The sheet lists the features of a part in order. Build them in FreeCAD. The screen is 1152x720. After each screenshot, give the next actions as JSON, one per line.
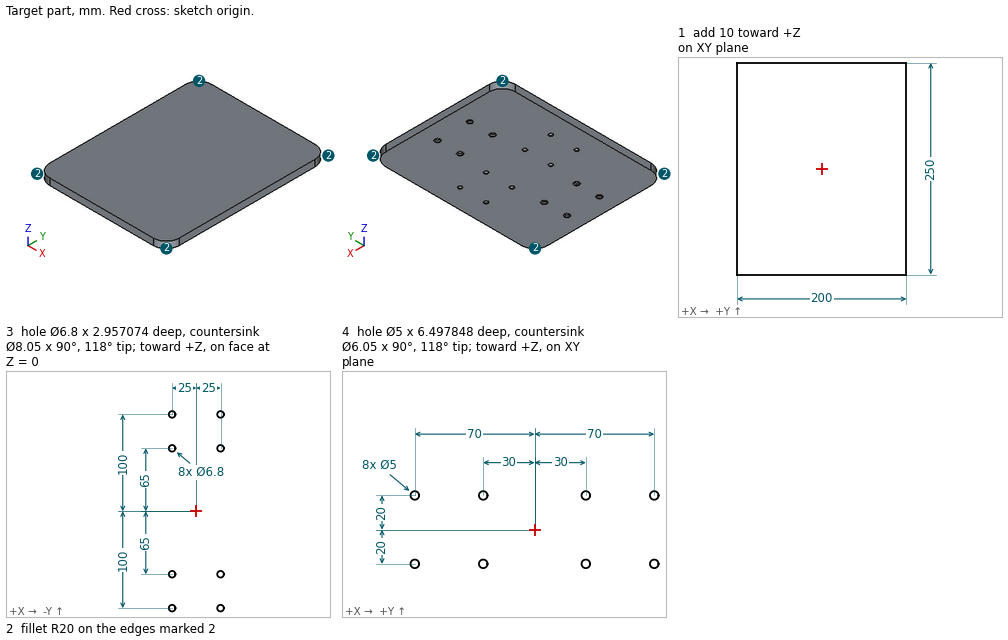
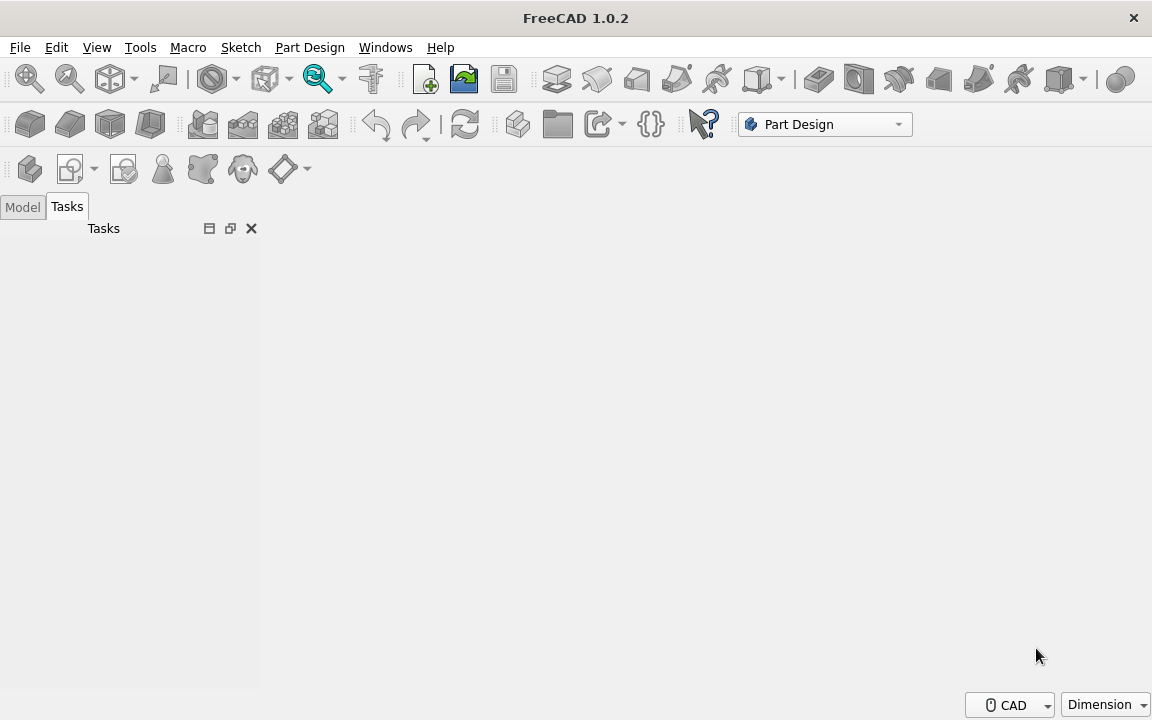
{"action": "left_click", "coordinate": [424, 80]}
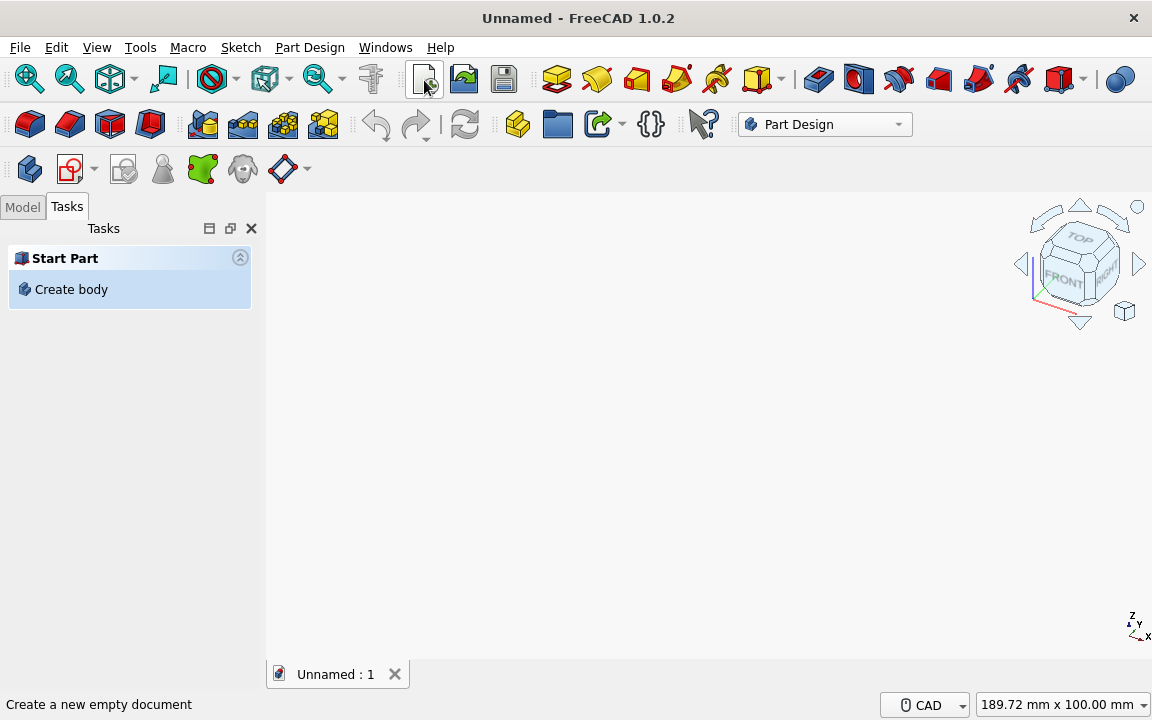
{"action": "left_click", "coordinate": [70, 170]}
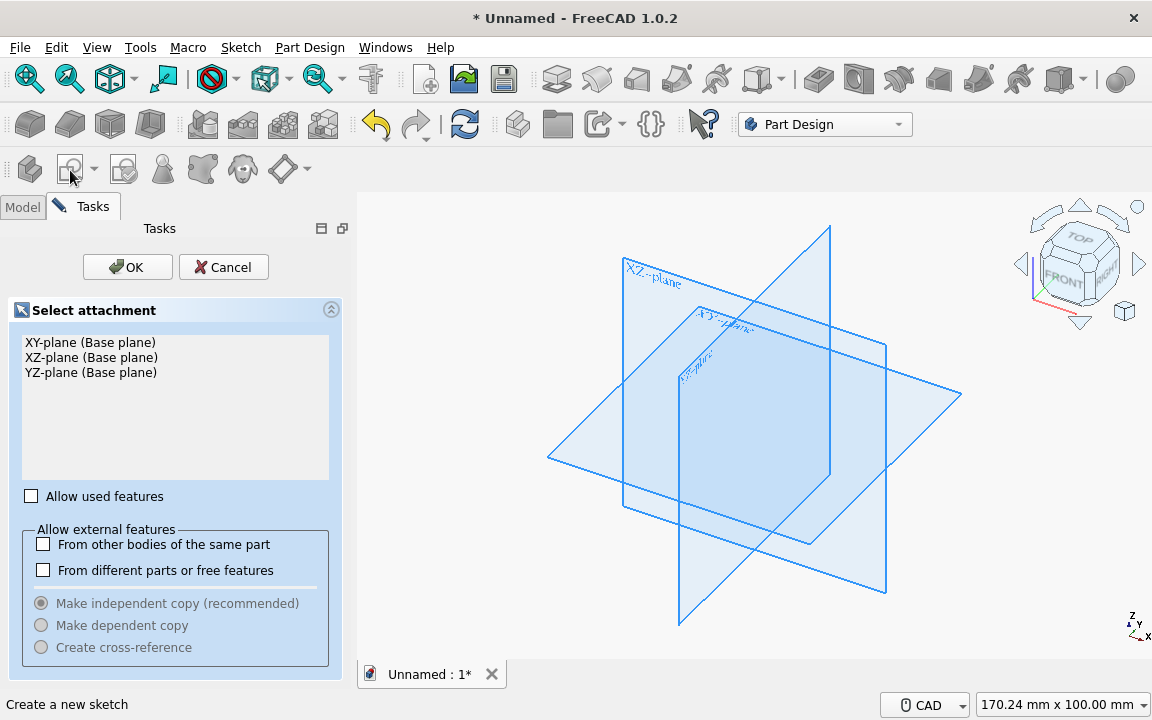
{"action": "left_click", "coordinate": [82, 342]}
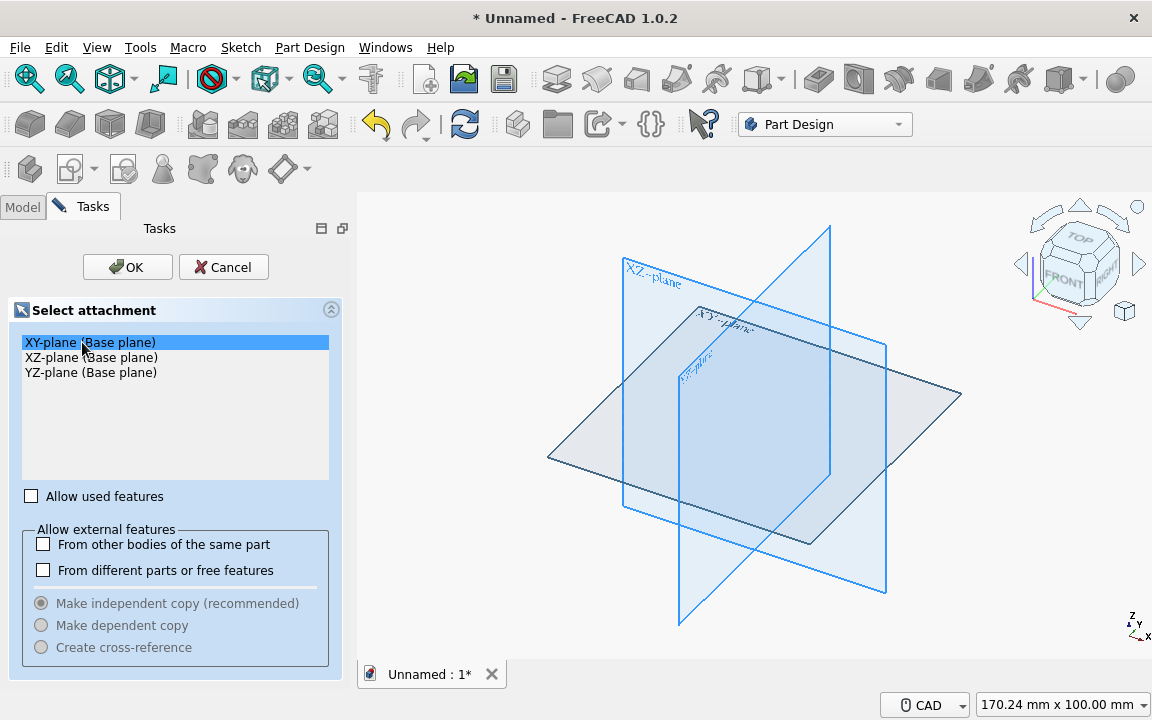
{"action": "left_click", "coordinate": [128, 267]}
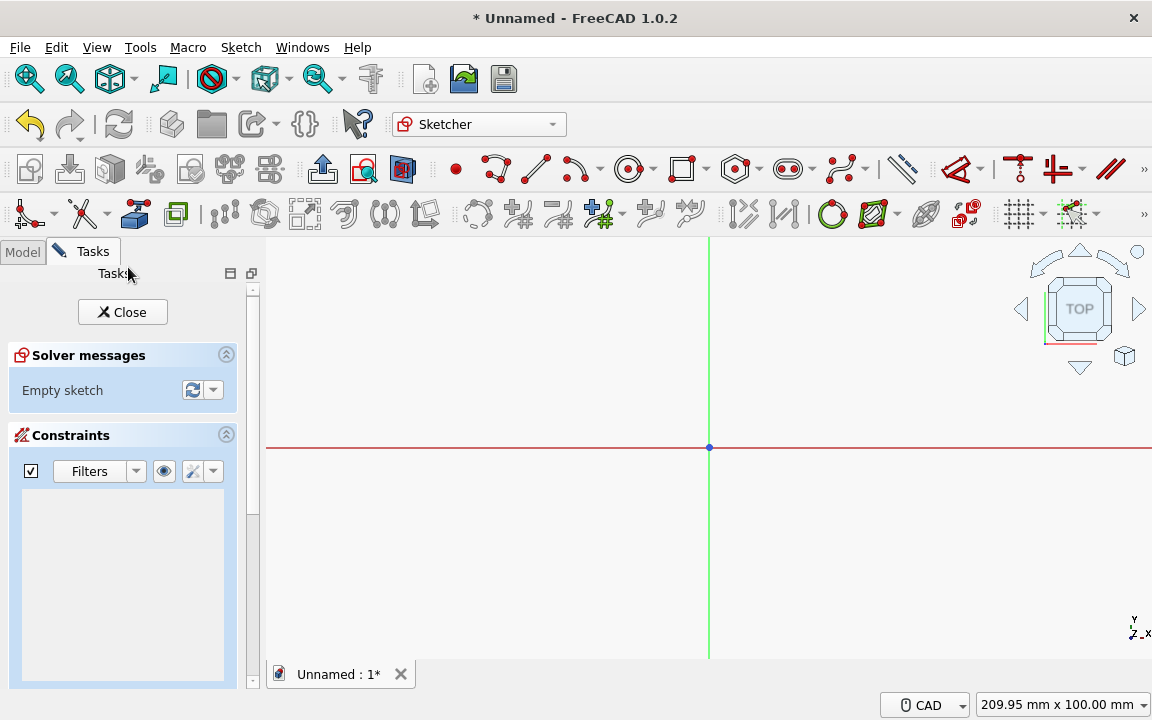
{"action": "scroll", "coordinate": [618, 448], "scroll_direction": "down", "scroll_amount": 7}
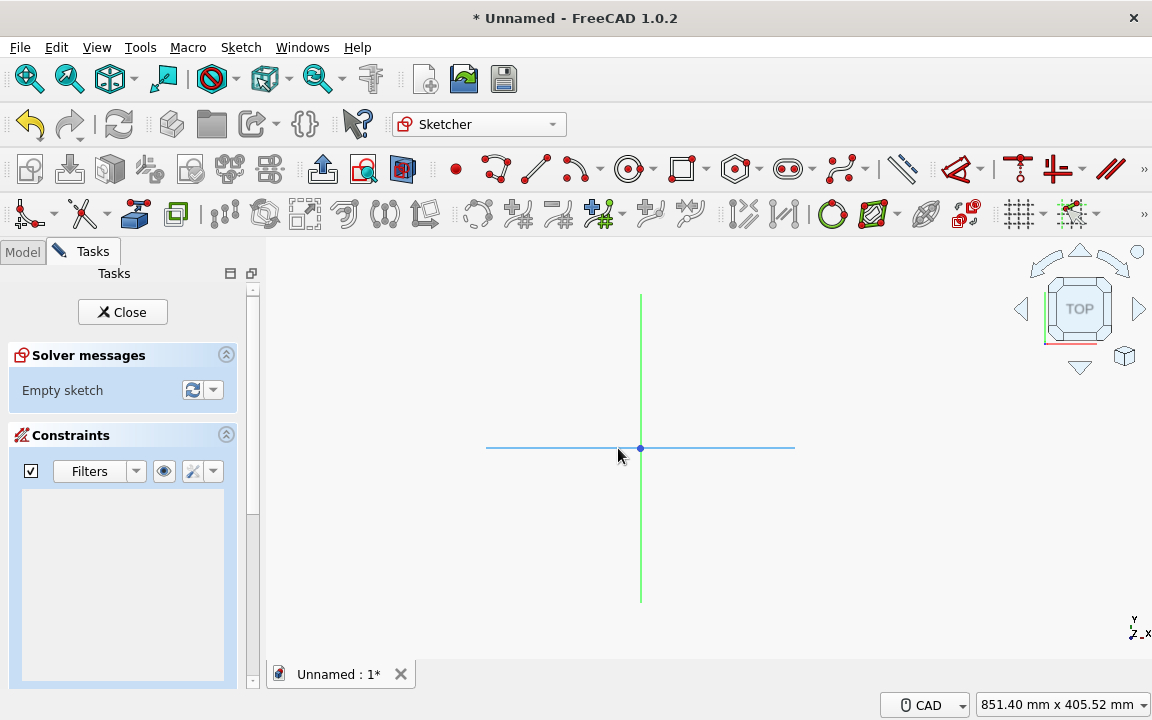
{"action": "key", "text": "g v"}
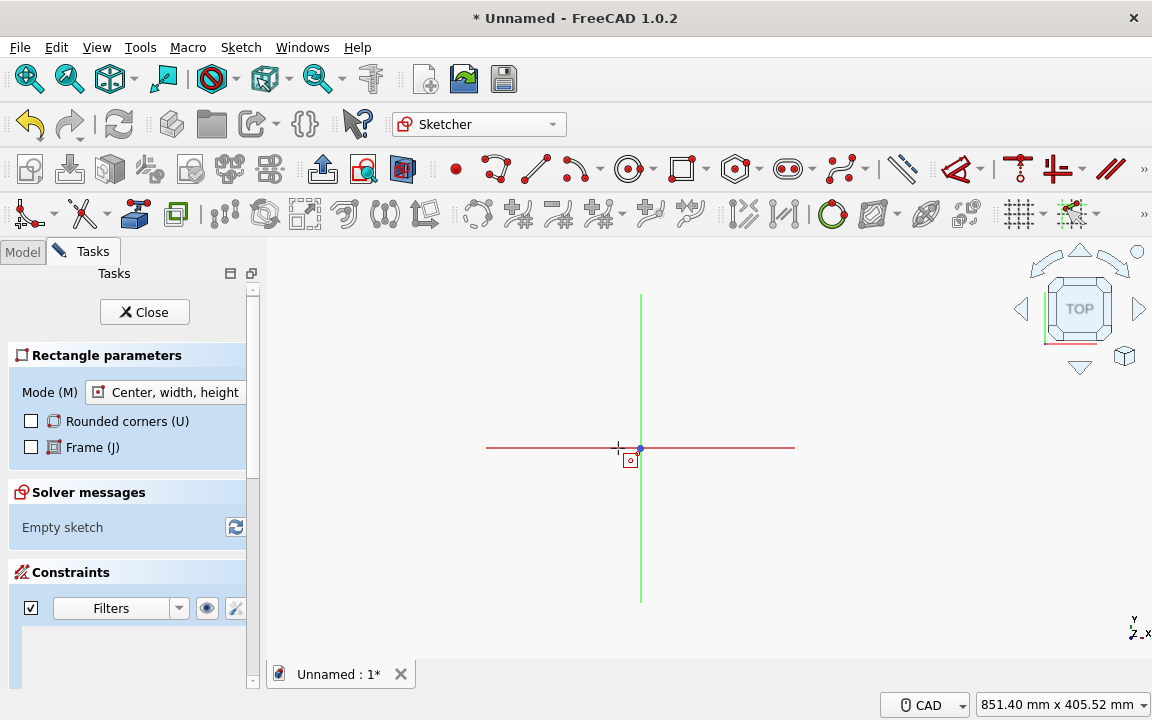
{"action": "left_click", "coordinate": [641, 448]}
{"action": "mouse_move", "coordinate": [745, 318]}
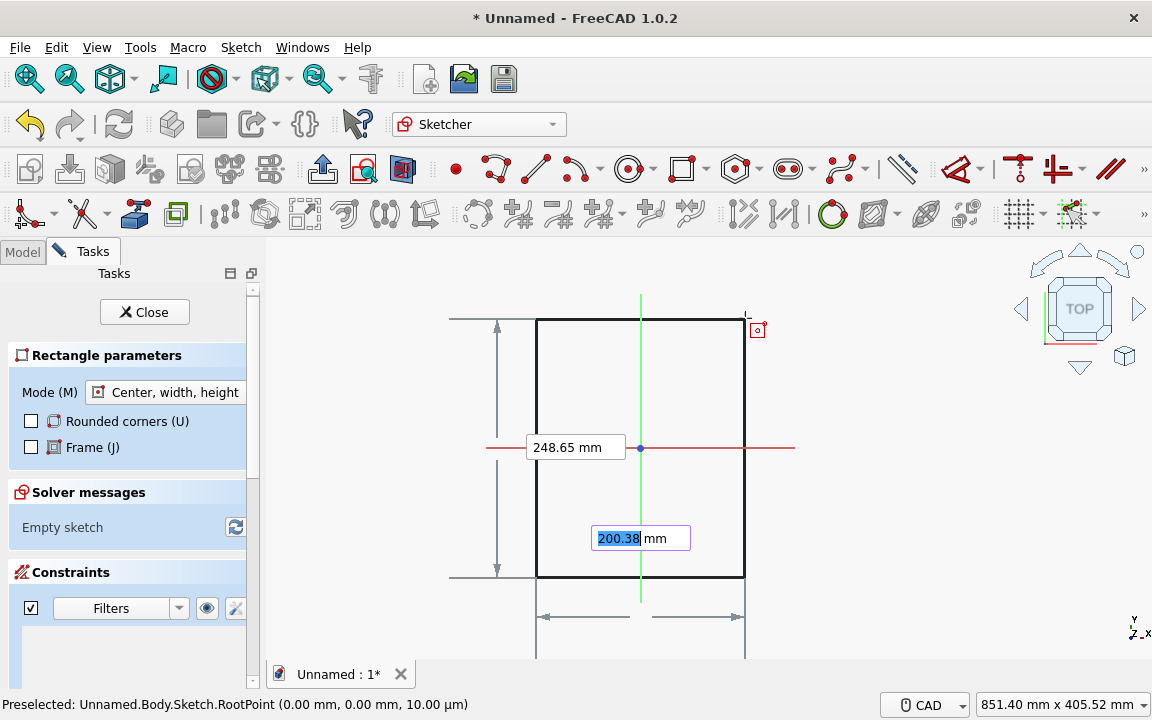
{"action": "type", "text": "200"}
{"action": "key", "text": "Tab"}
{"action": "type", "text": "250"}
{"action": "key", "text": "Return"}
{"action": "key", "text": "Escape"}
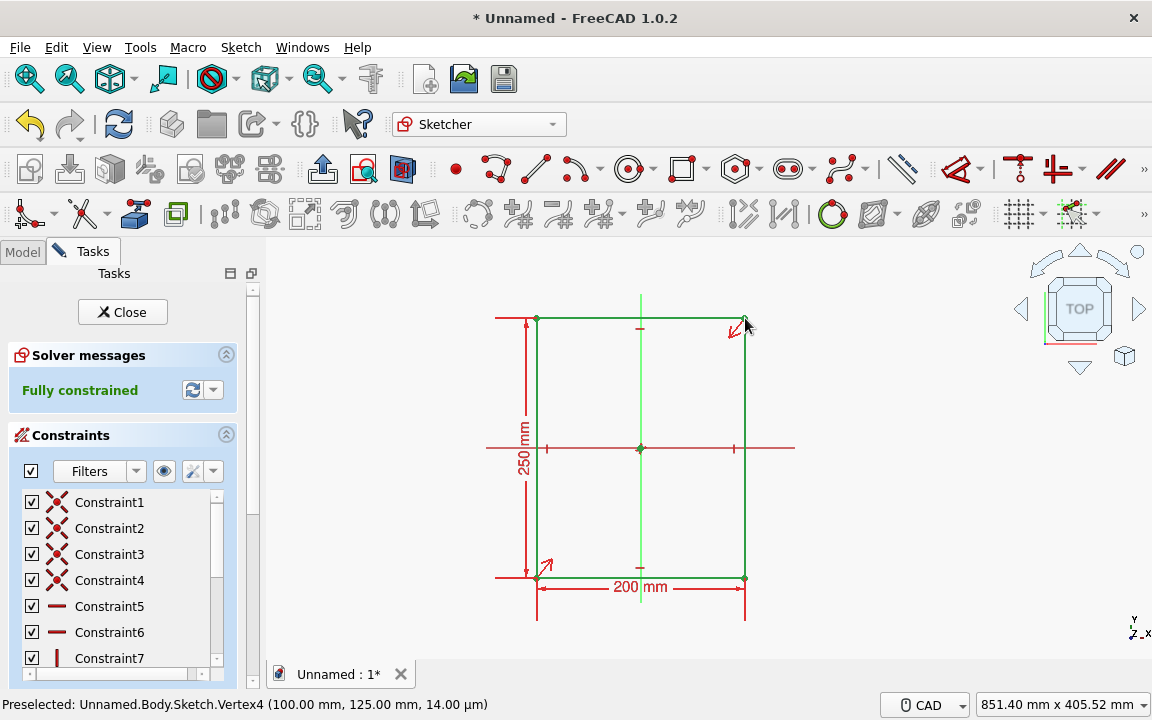
{"action": "left_click", "coordinate": [123, 312]}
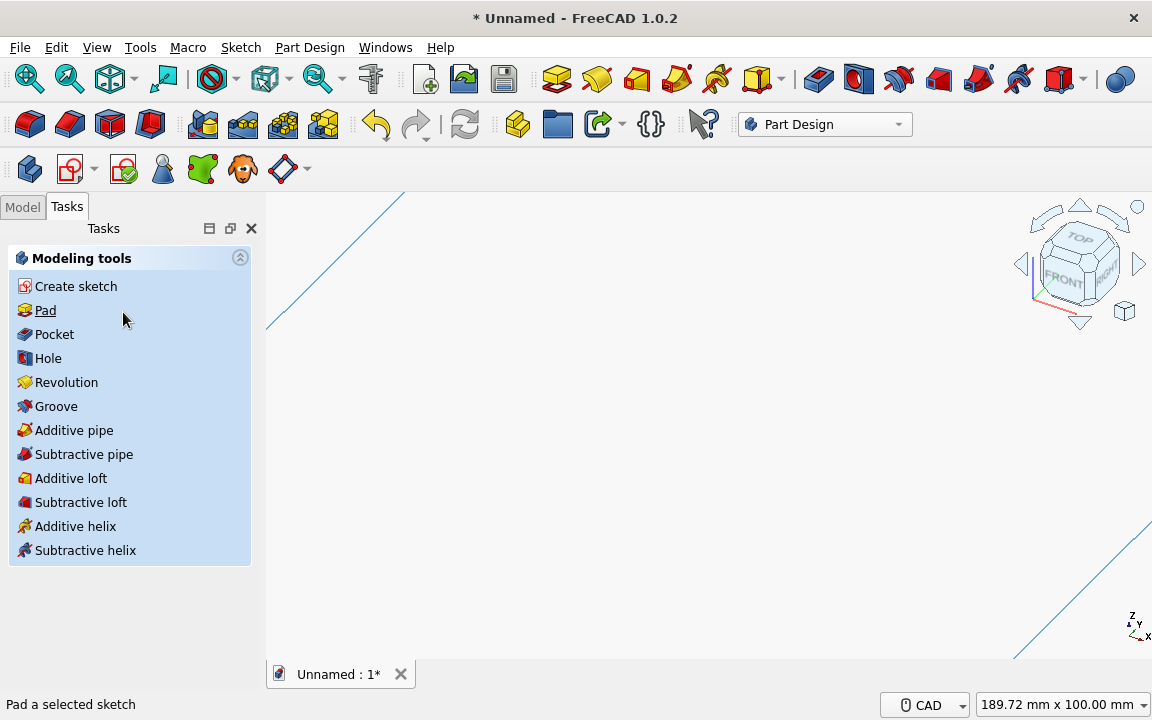
{"action": "left_click", "coordinate": [558, 80]}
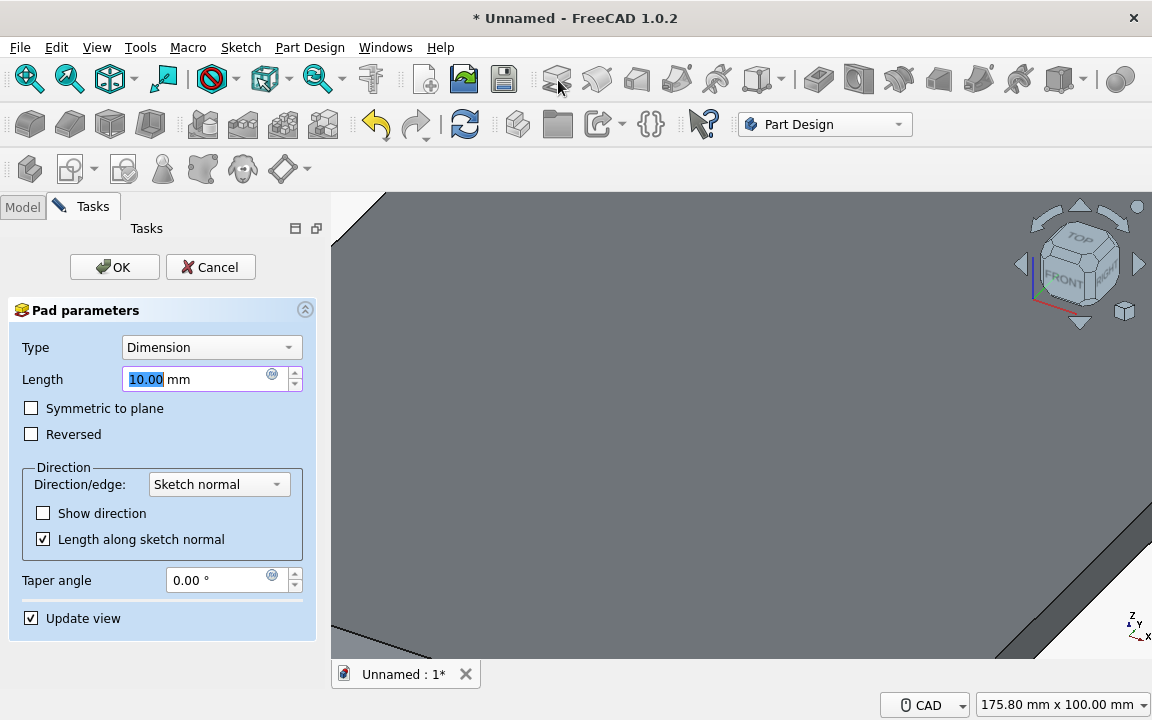
{"action": "type", "text": "10"}
{"action": "key", "text": "Tab"}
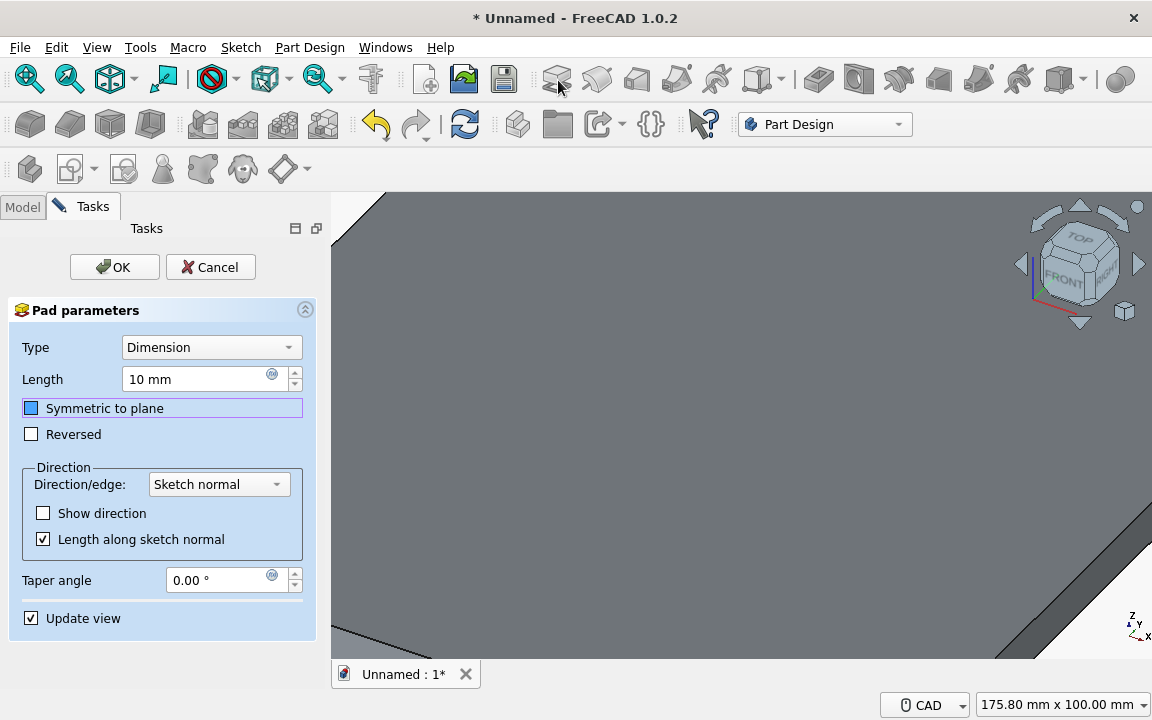
{"action": "left_click", "coordinate": [115, 267]}